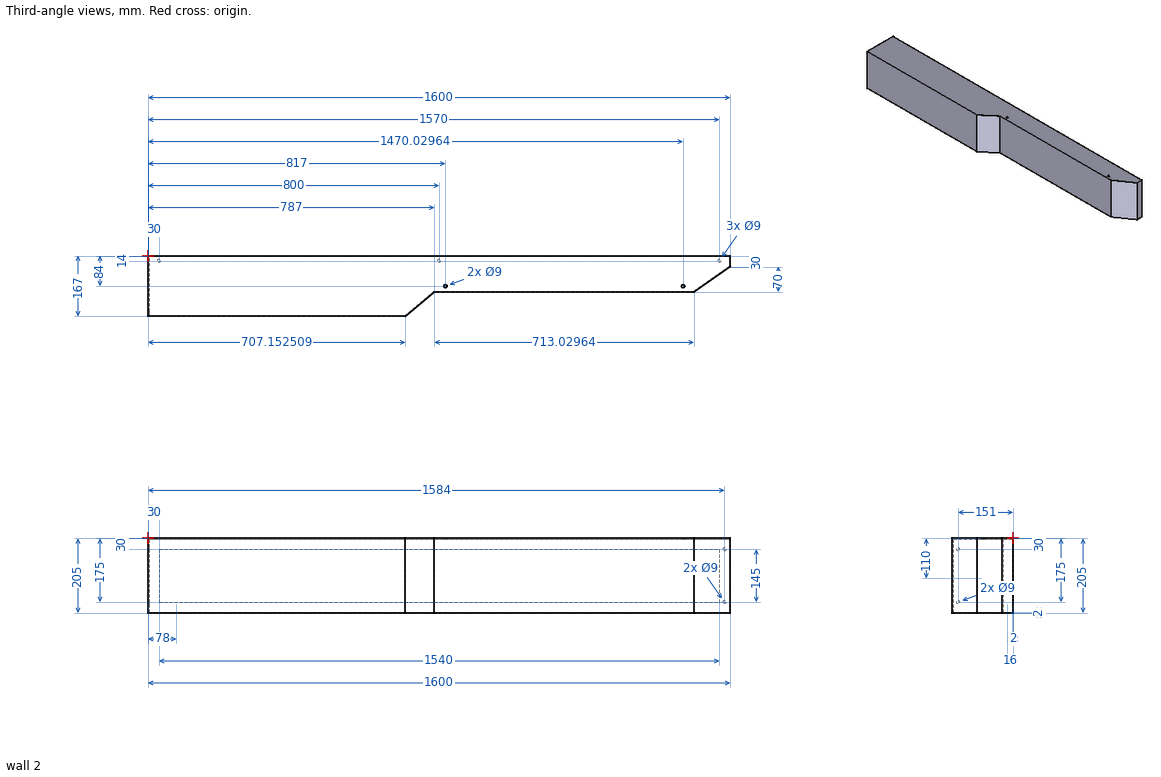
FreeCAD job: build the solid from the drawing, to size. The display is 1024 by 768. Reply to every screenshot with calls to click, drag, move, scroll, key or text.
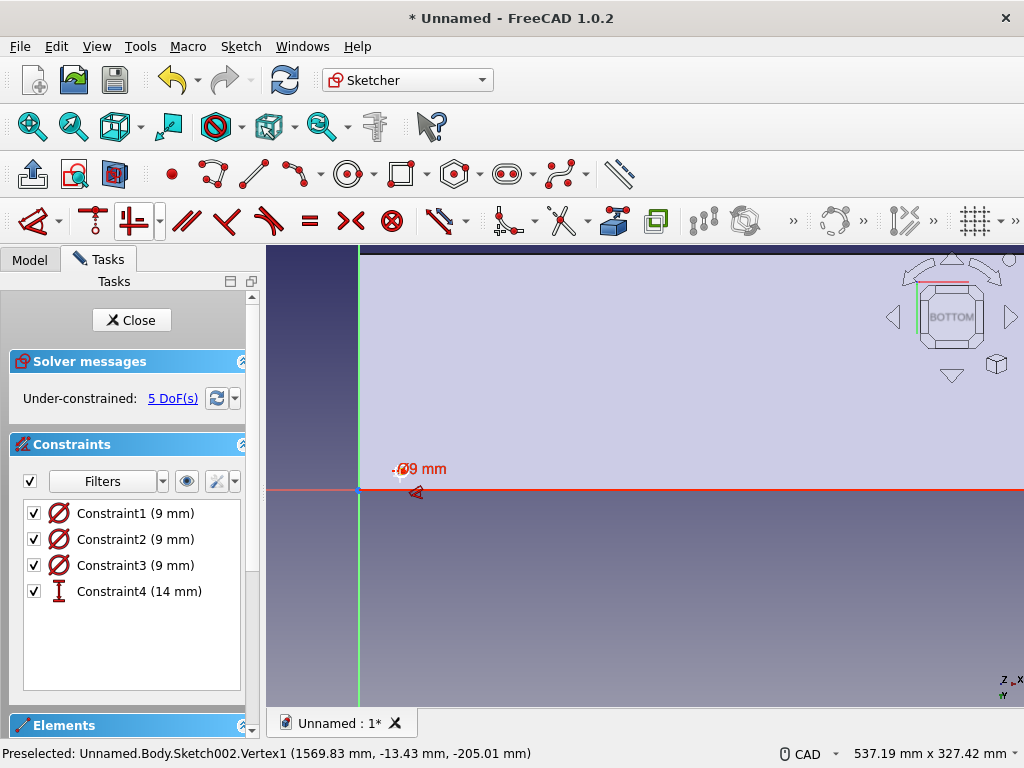
click(402, 471)
click(380, 524)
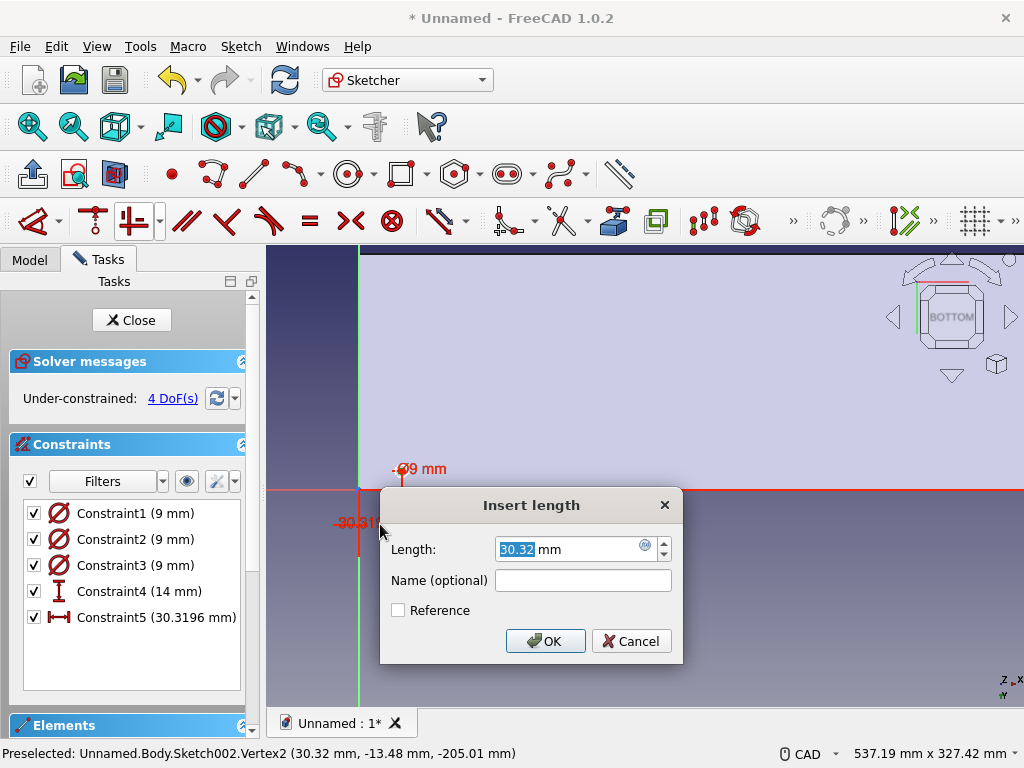
text(30)
key(Return)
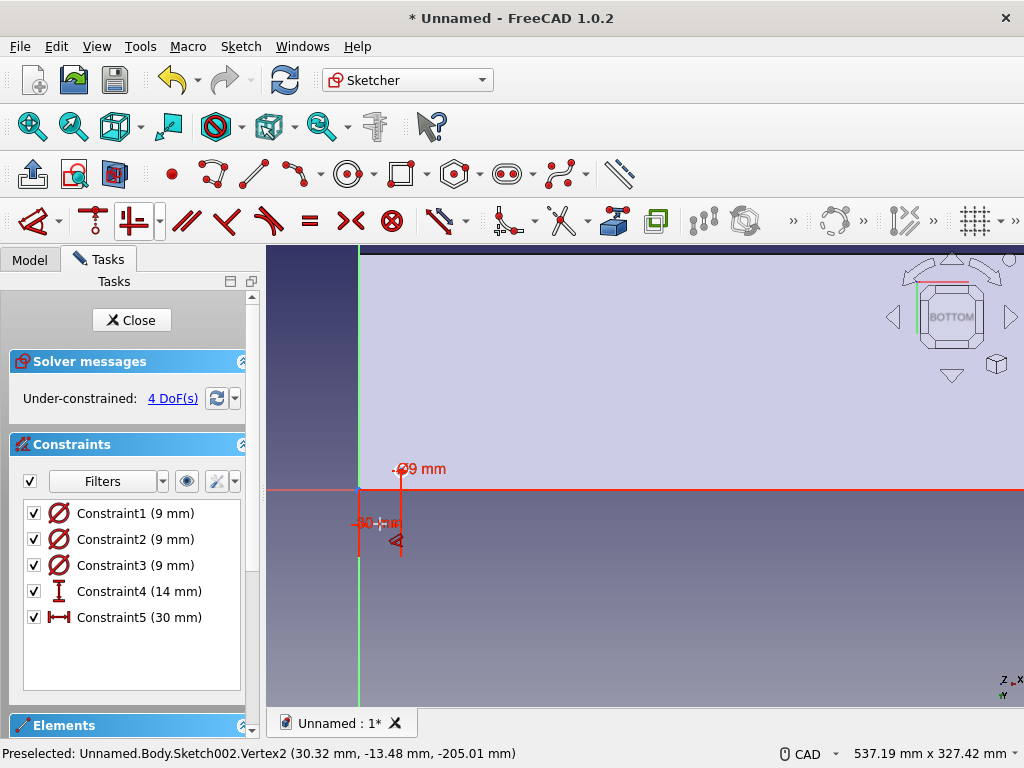
scroll(401, 471, up, 4)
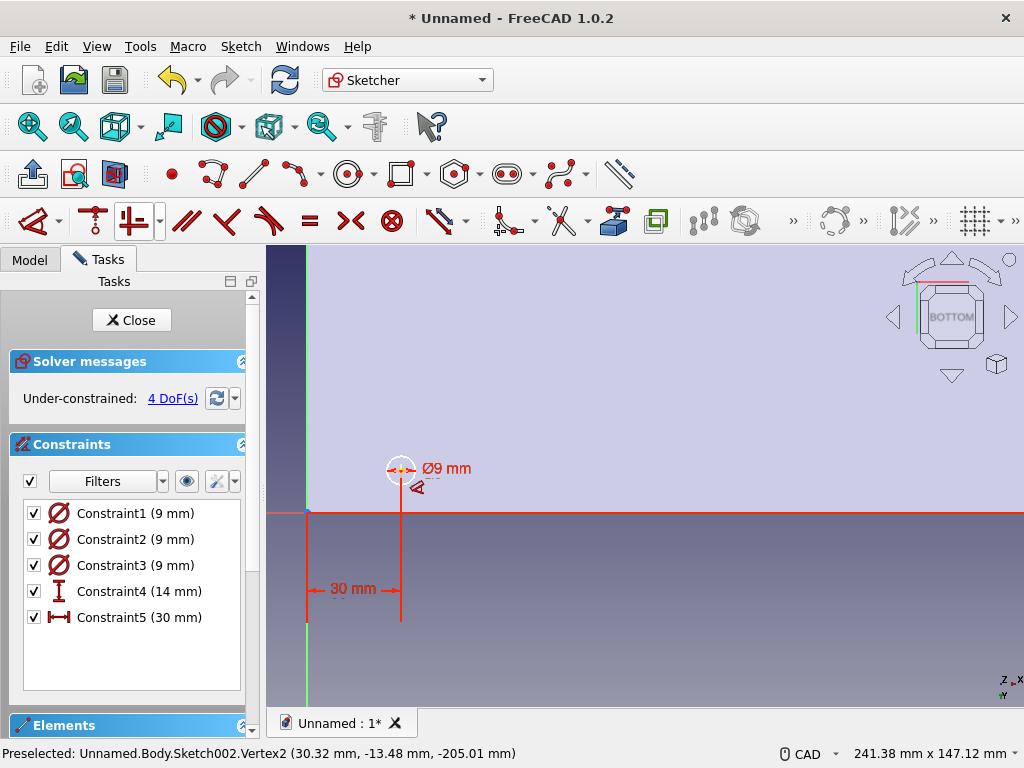
click(401, 471)
click(435, 492)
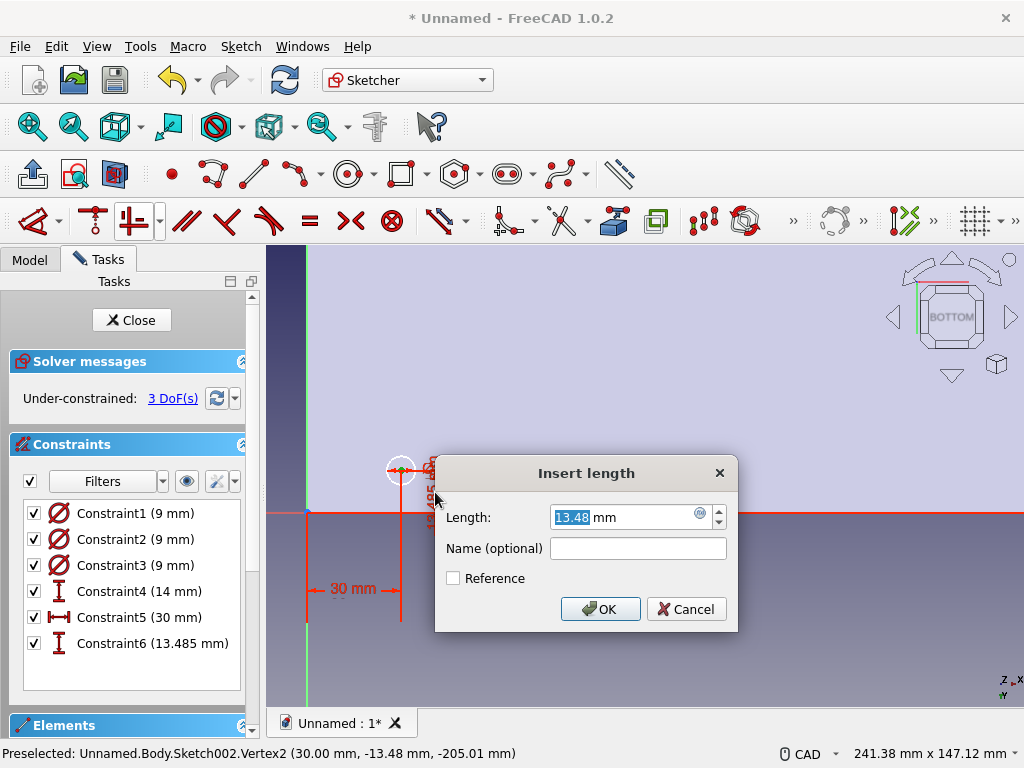
text(14)
key(Return)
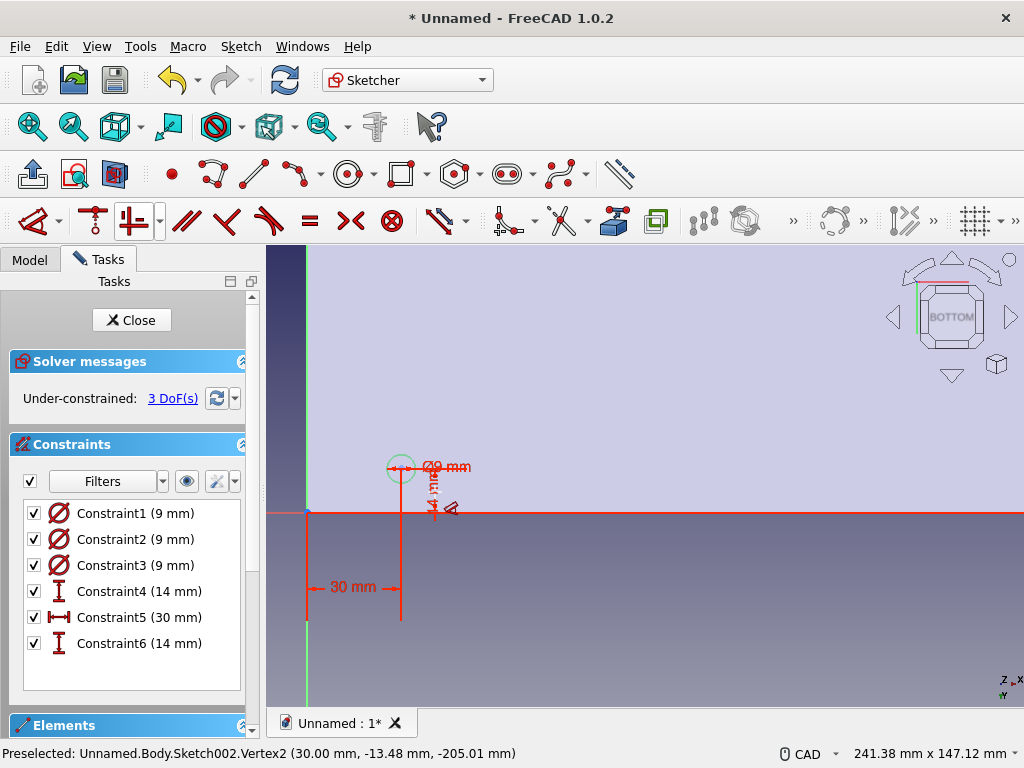
scroll(400, 475, down, 13)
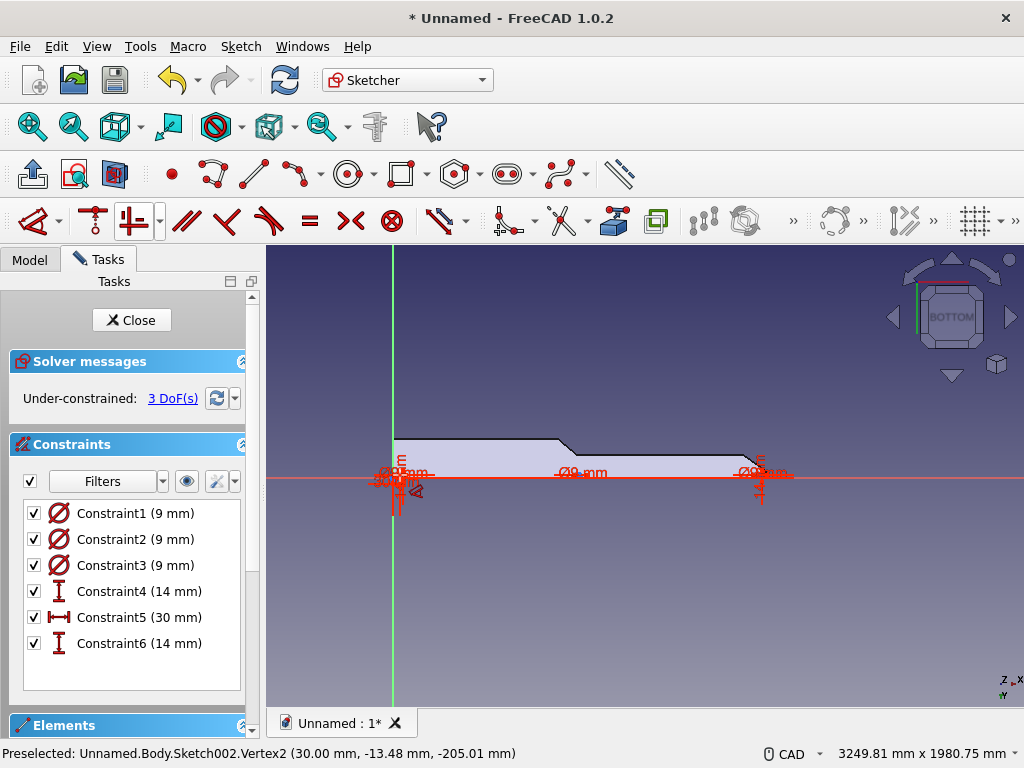
scroll(580, 475, up, 13)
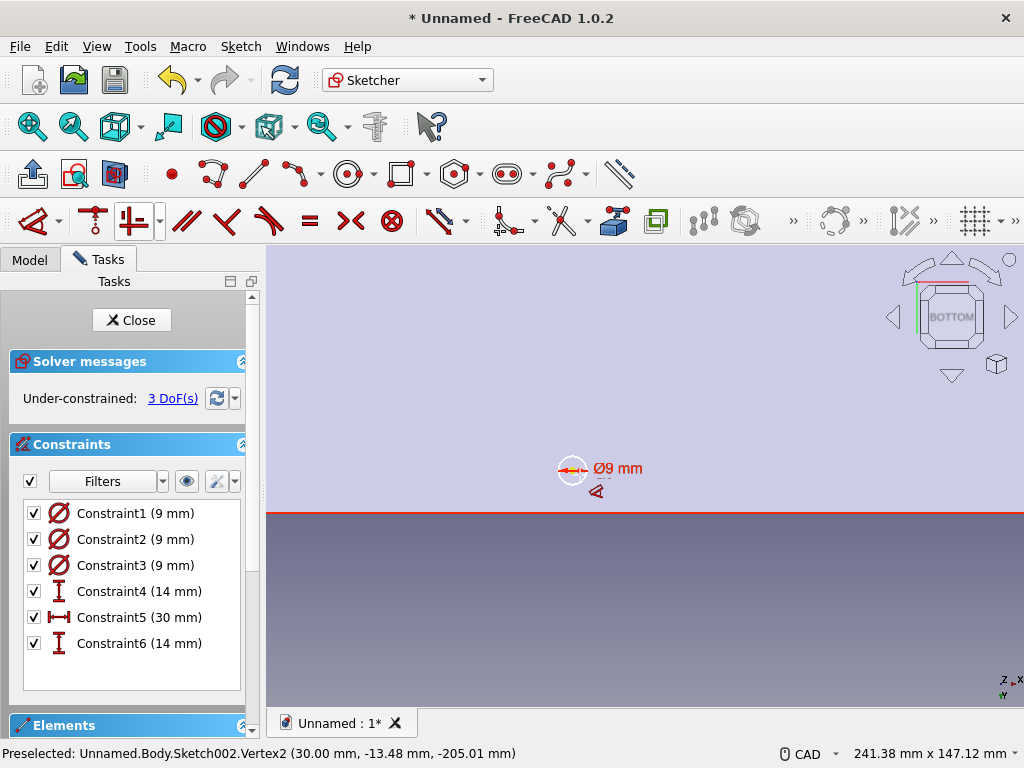
click(573, 471)
click(607, 492)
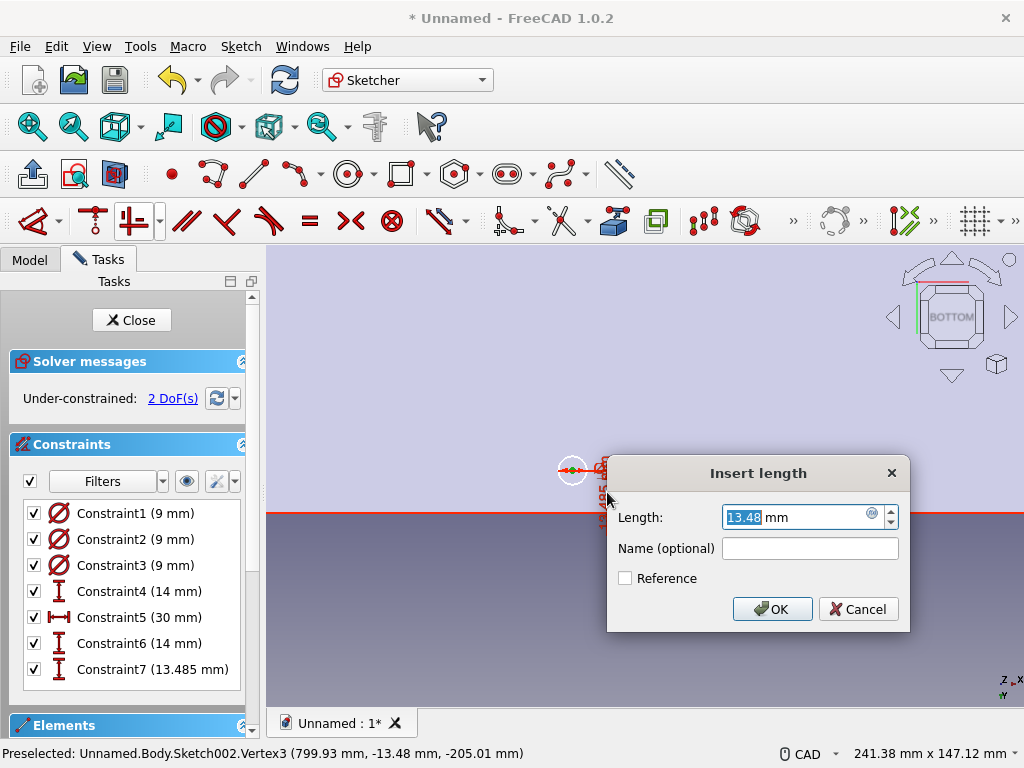
text(14)
key(Return)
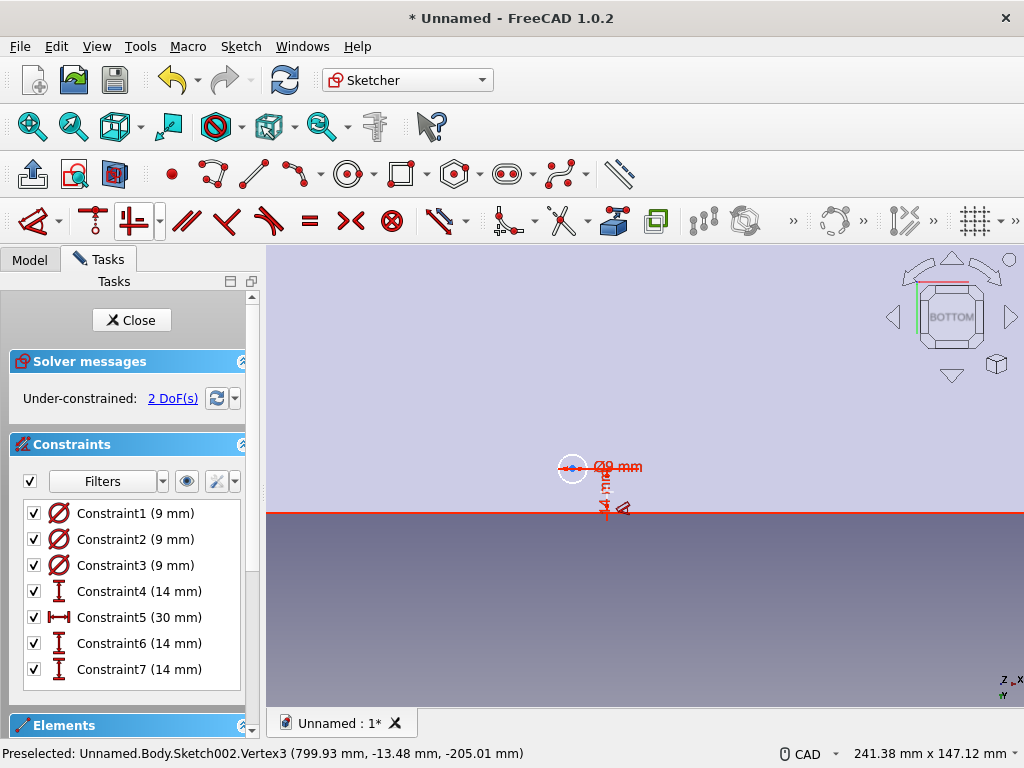
scroll(580, 475, down, 13)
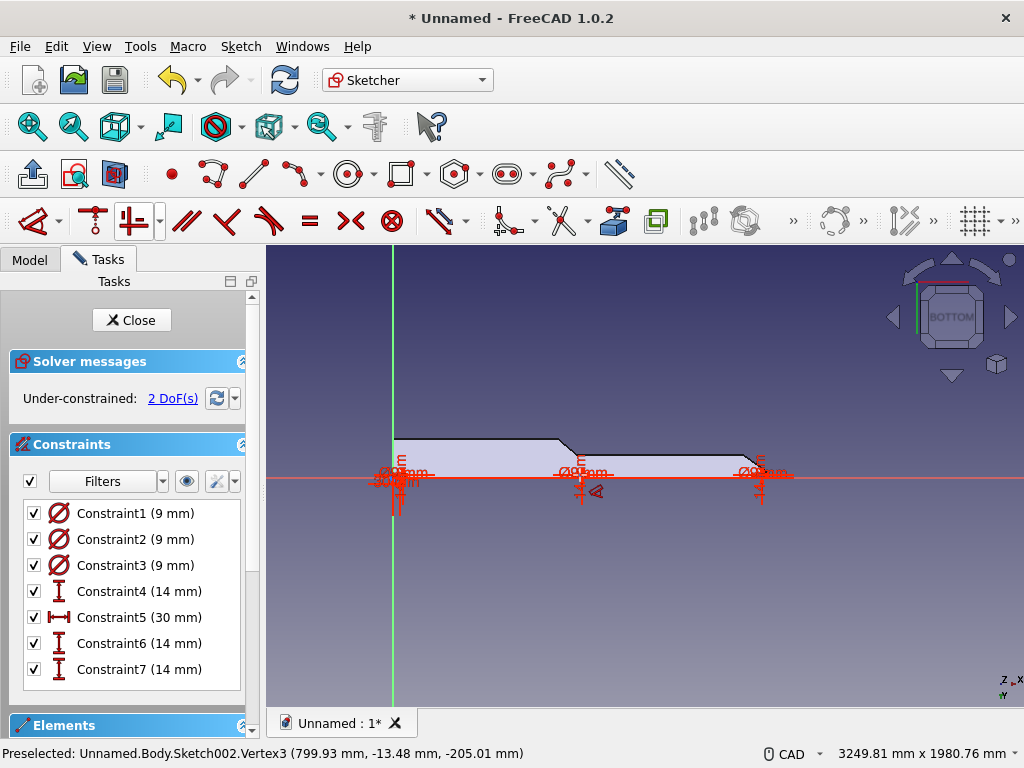
click(580, 475)
click(487, 512)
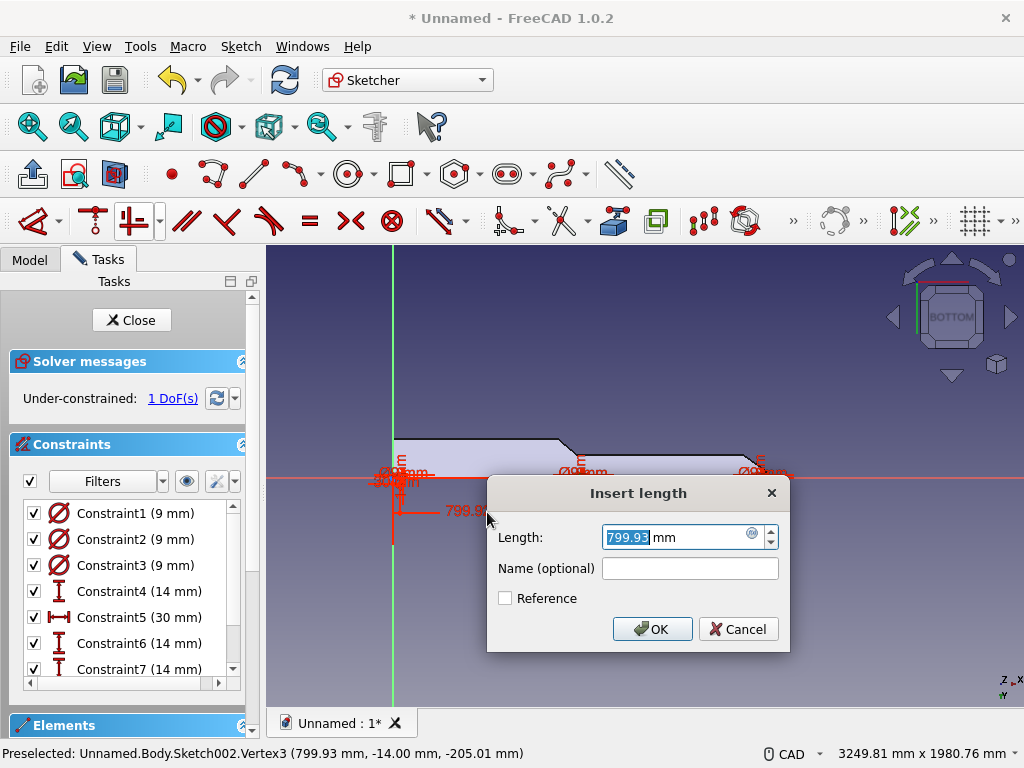
text(800)
key(Return)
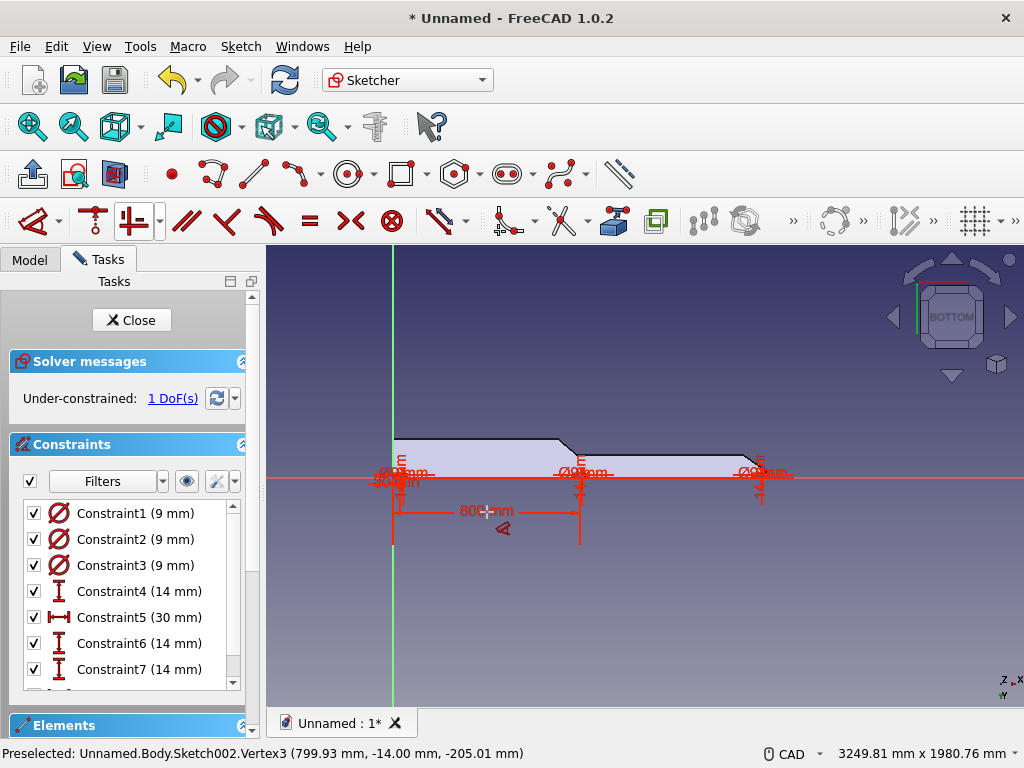
click(759, 475)
click(576, 512)